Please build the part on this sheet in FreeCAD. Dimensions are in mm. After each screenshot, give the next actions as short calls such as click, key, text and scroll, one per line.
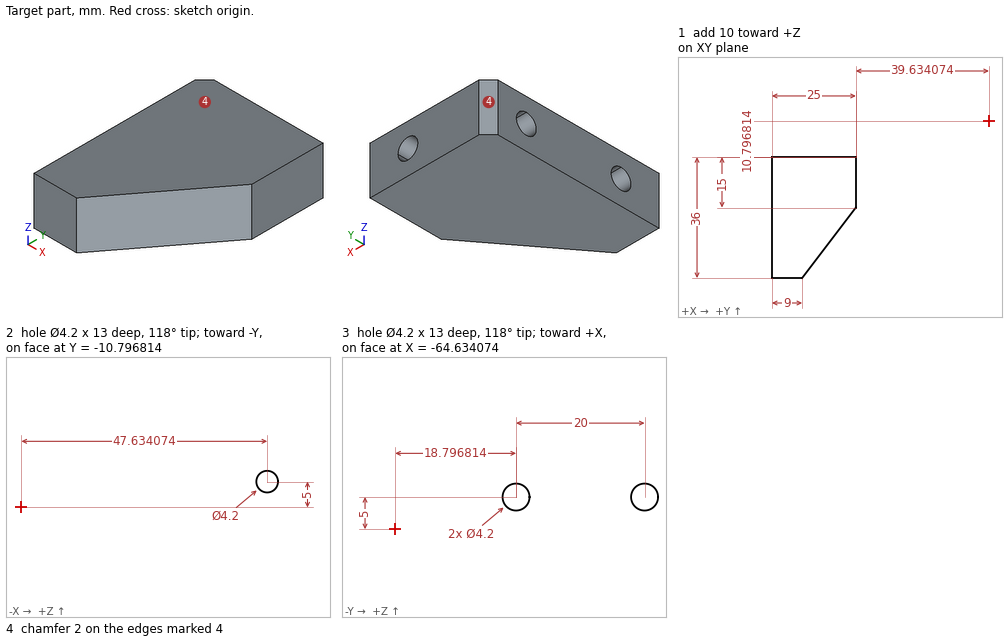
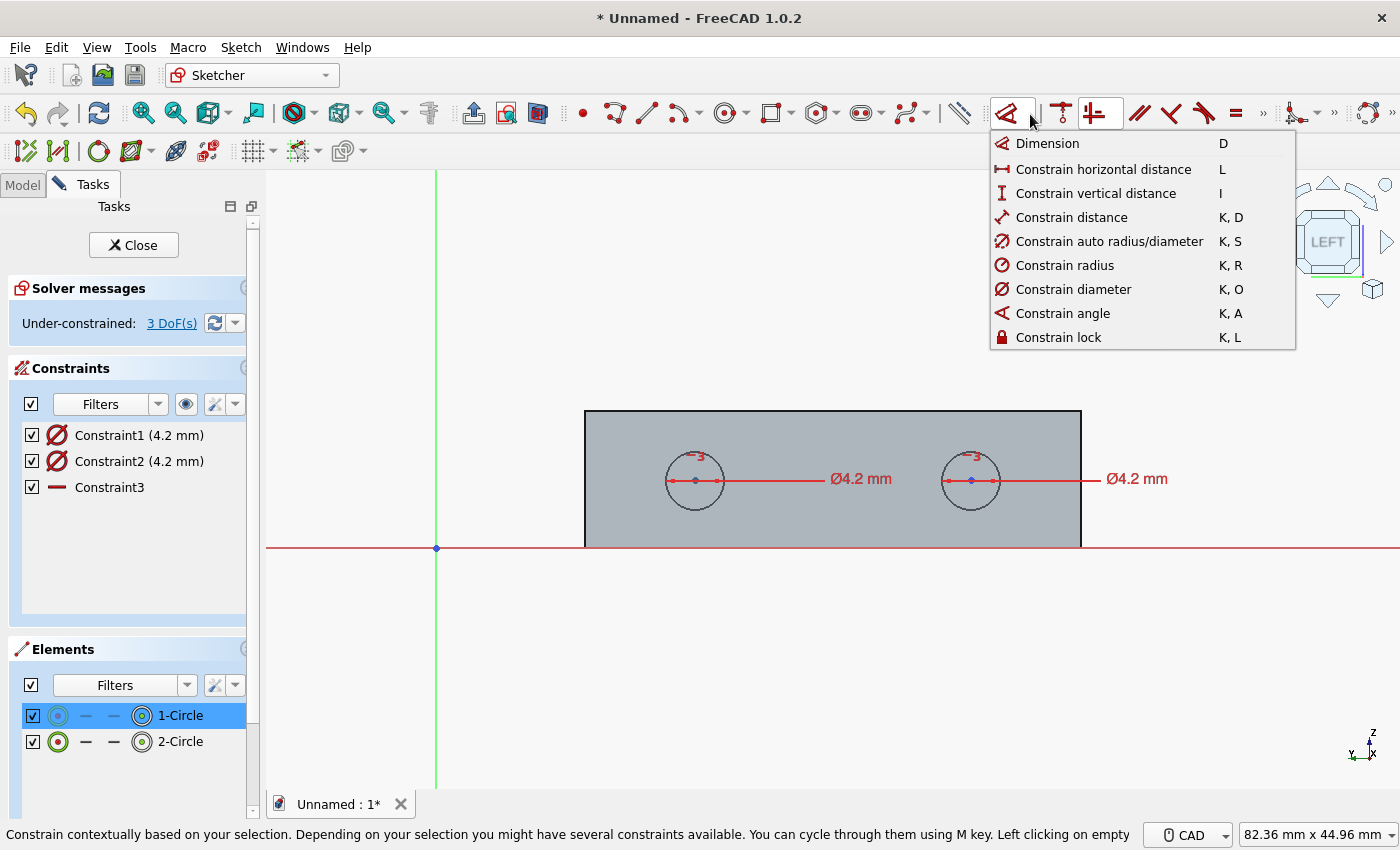
click(1143, 193)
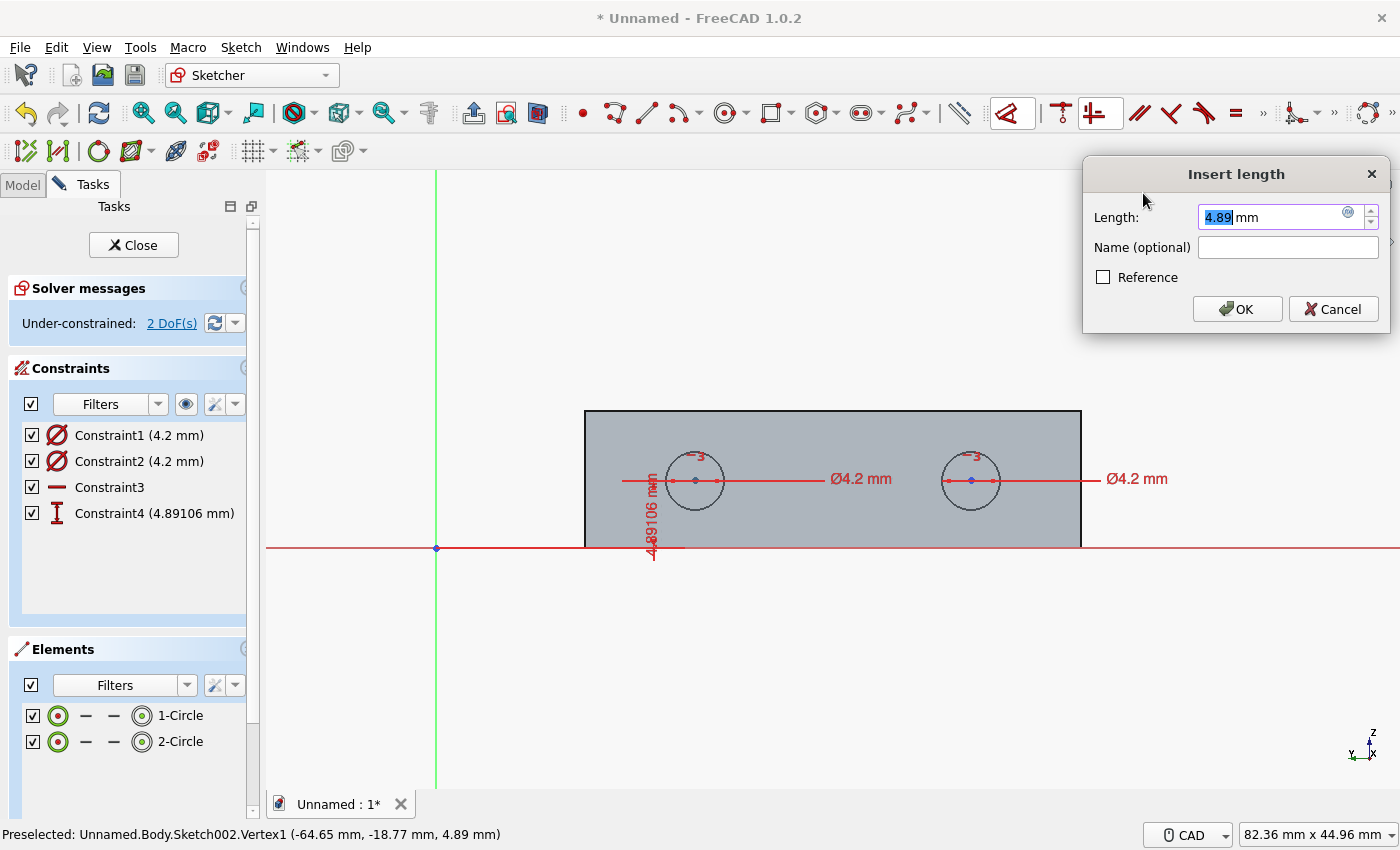
text(5)
key(Return)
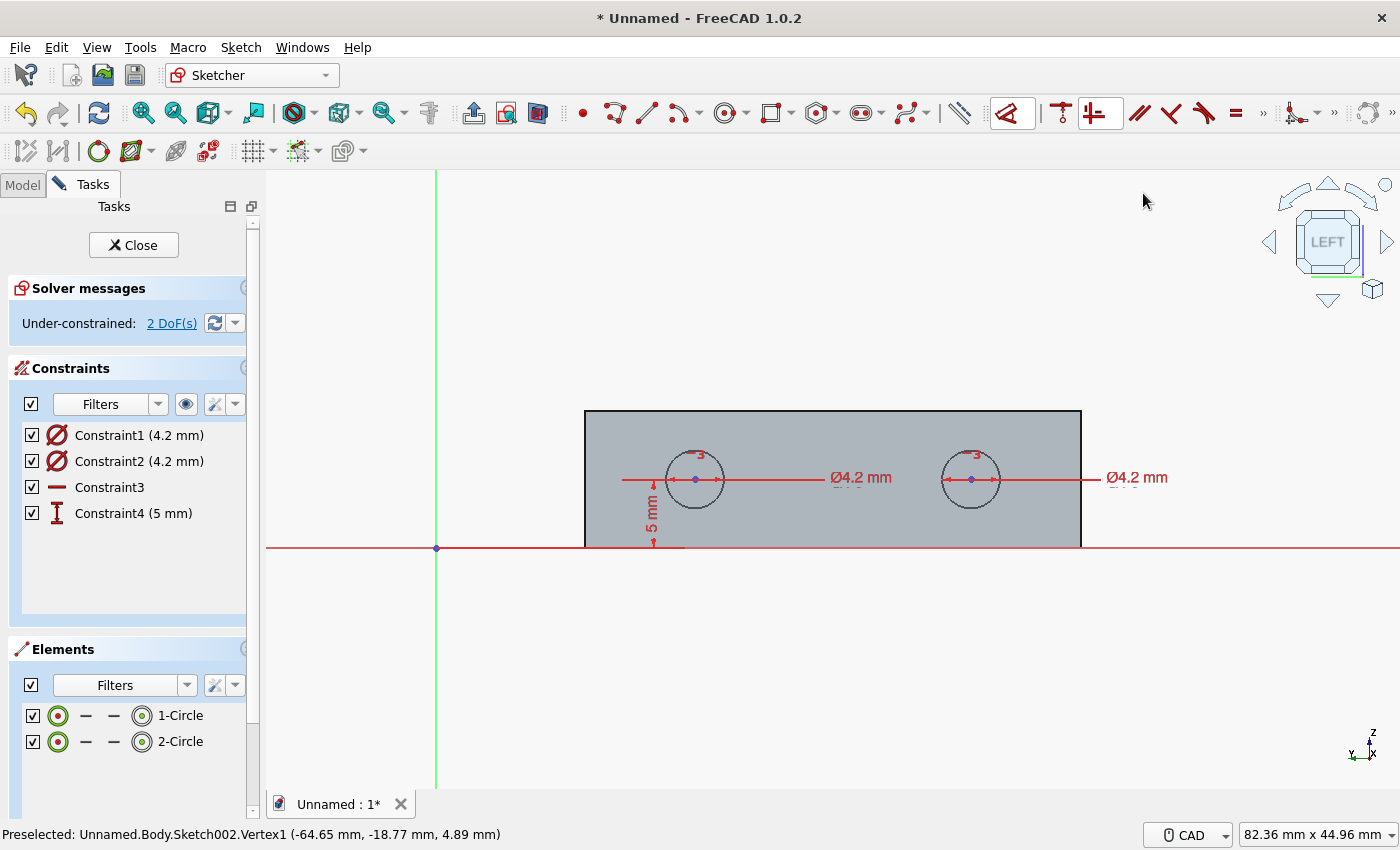
click(695, 480)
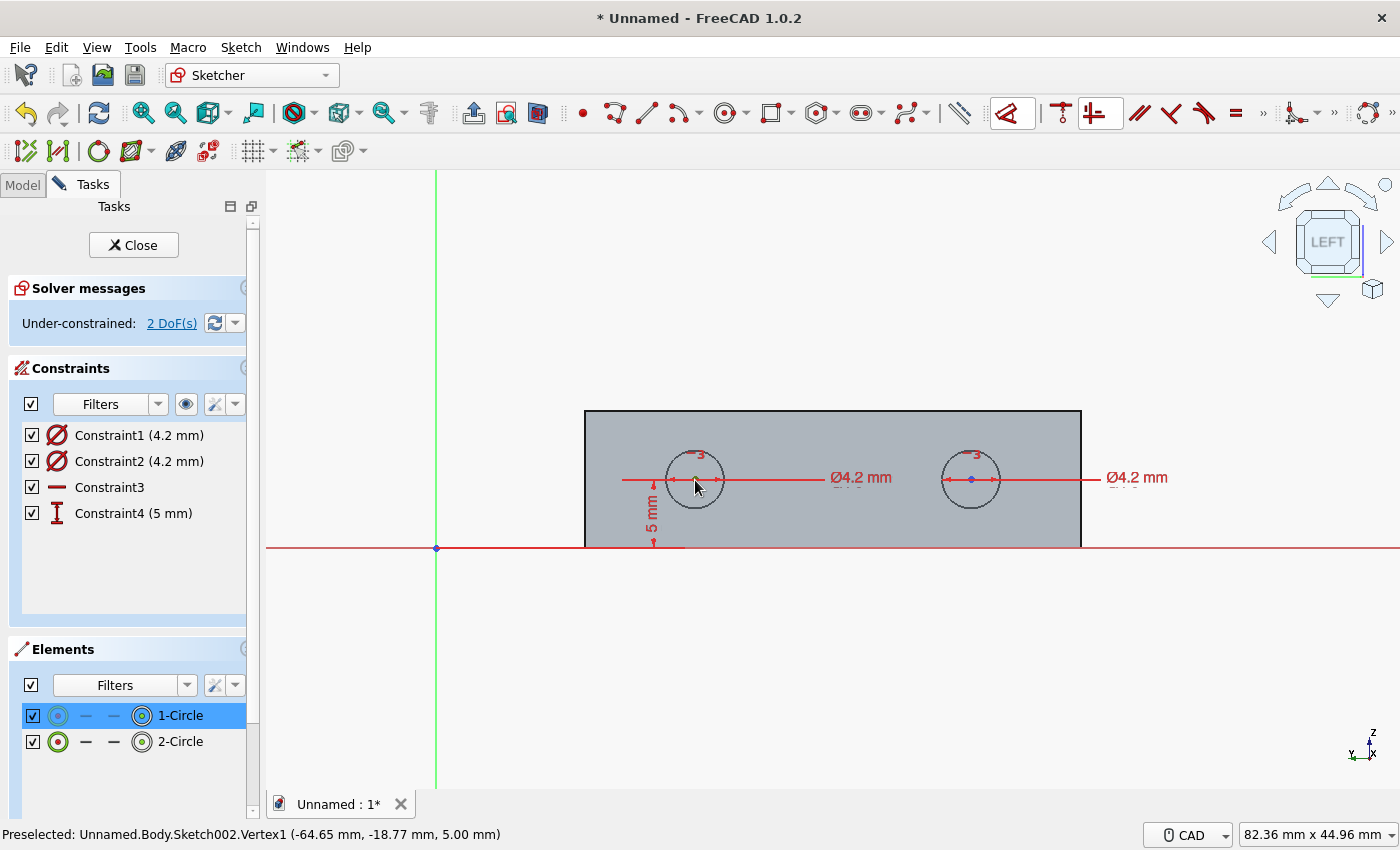
click(971, 480)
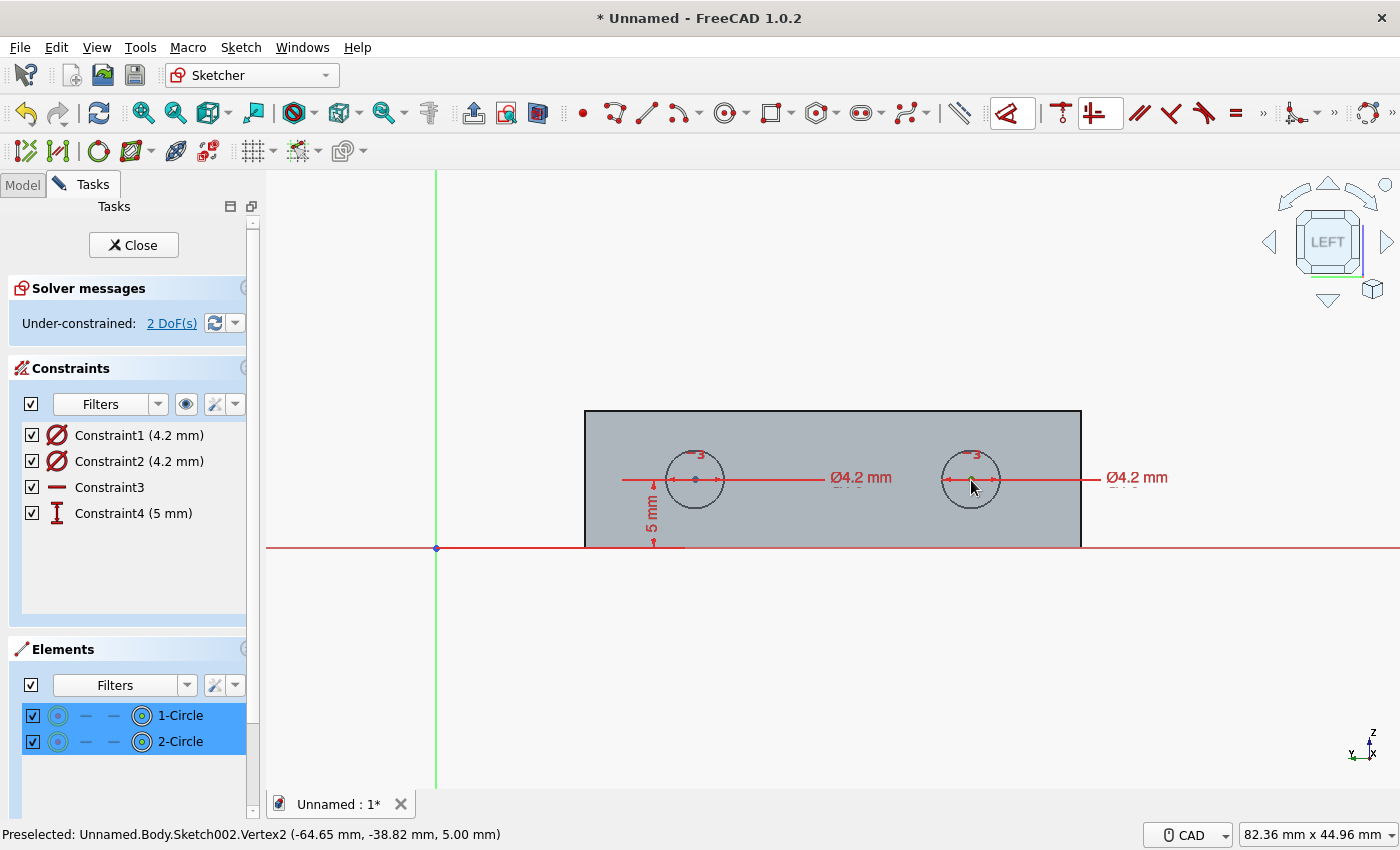
click(1030, 114)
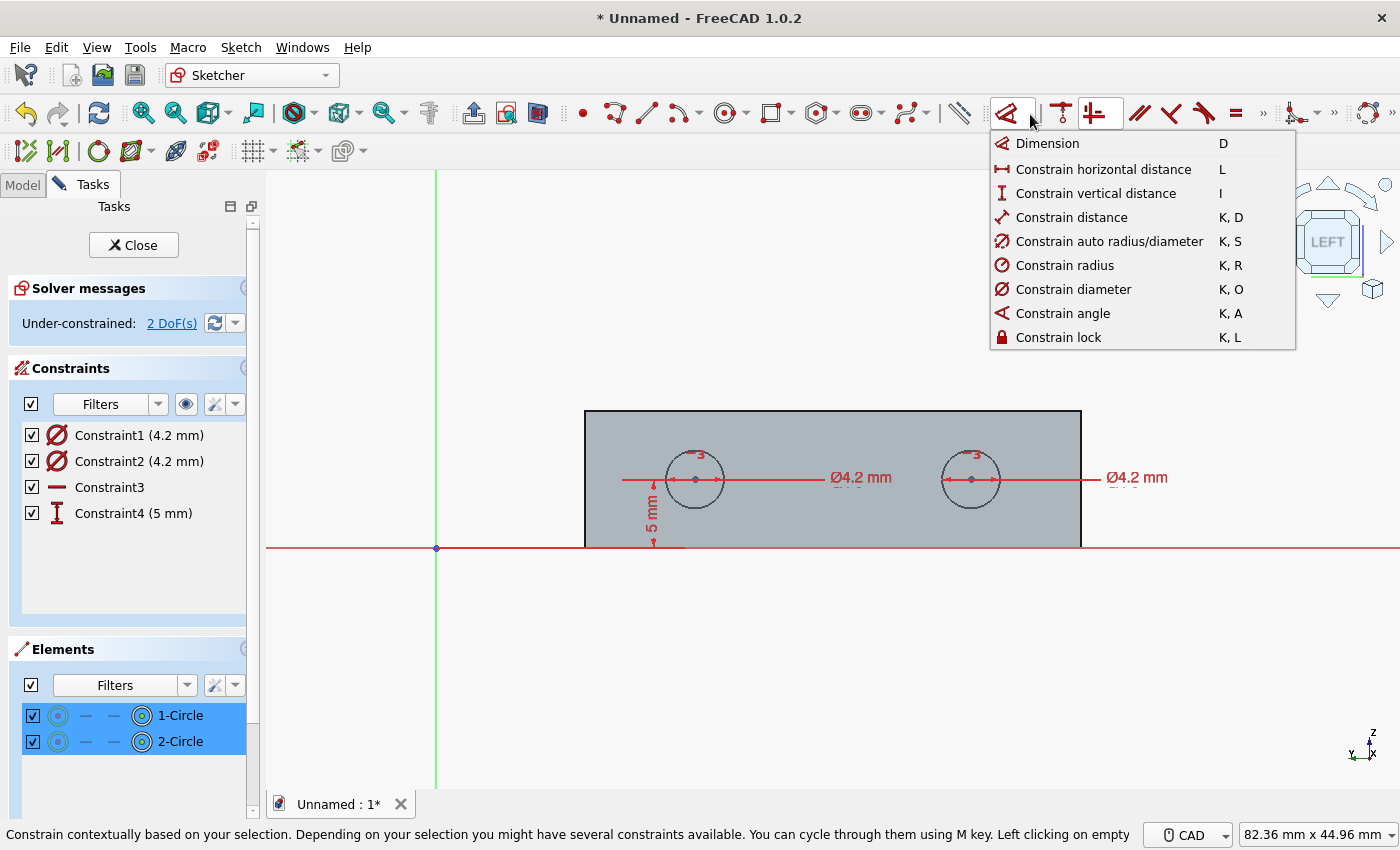
click(1143, 169)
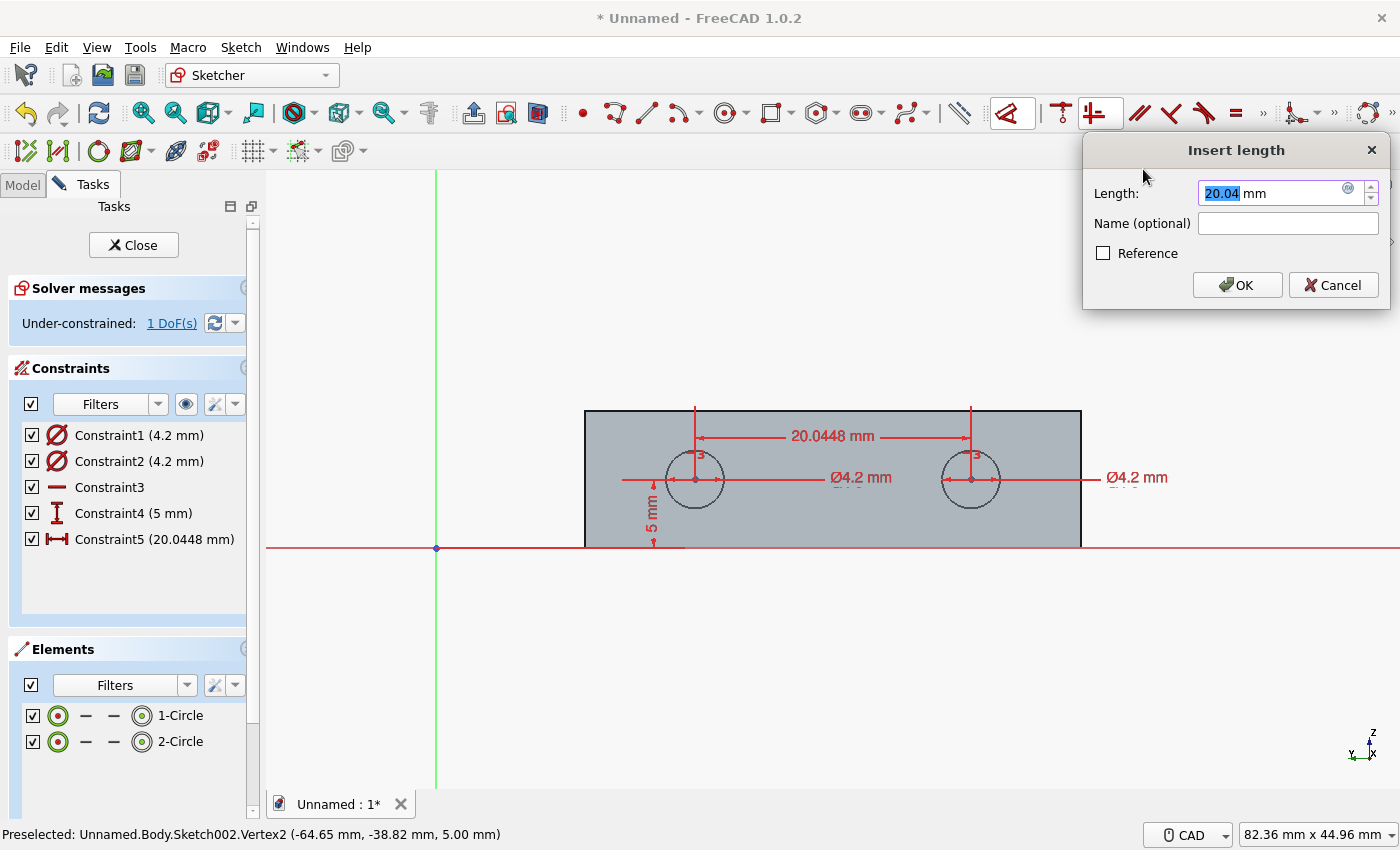
text(20)
key(Return)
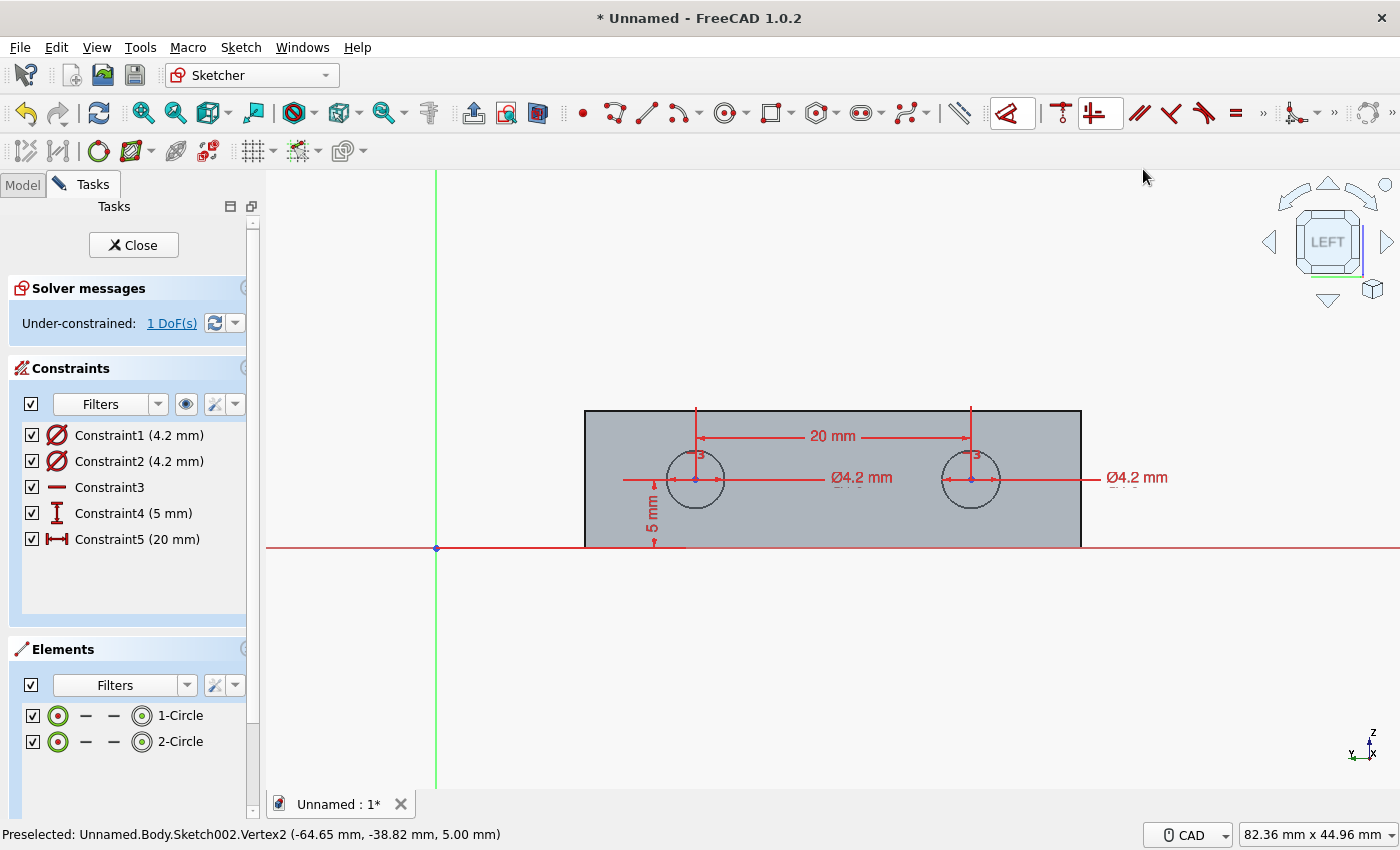
click(696, 480)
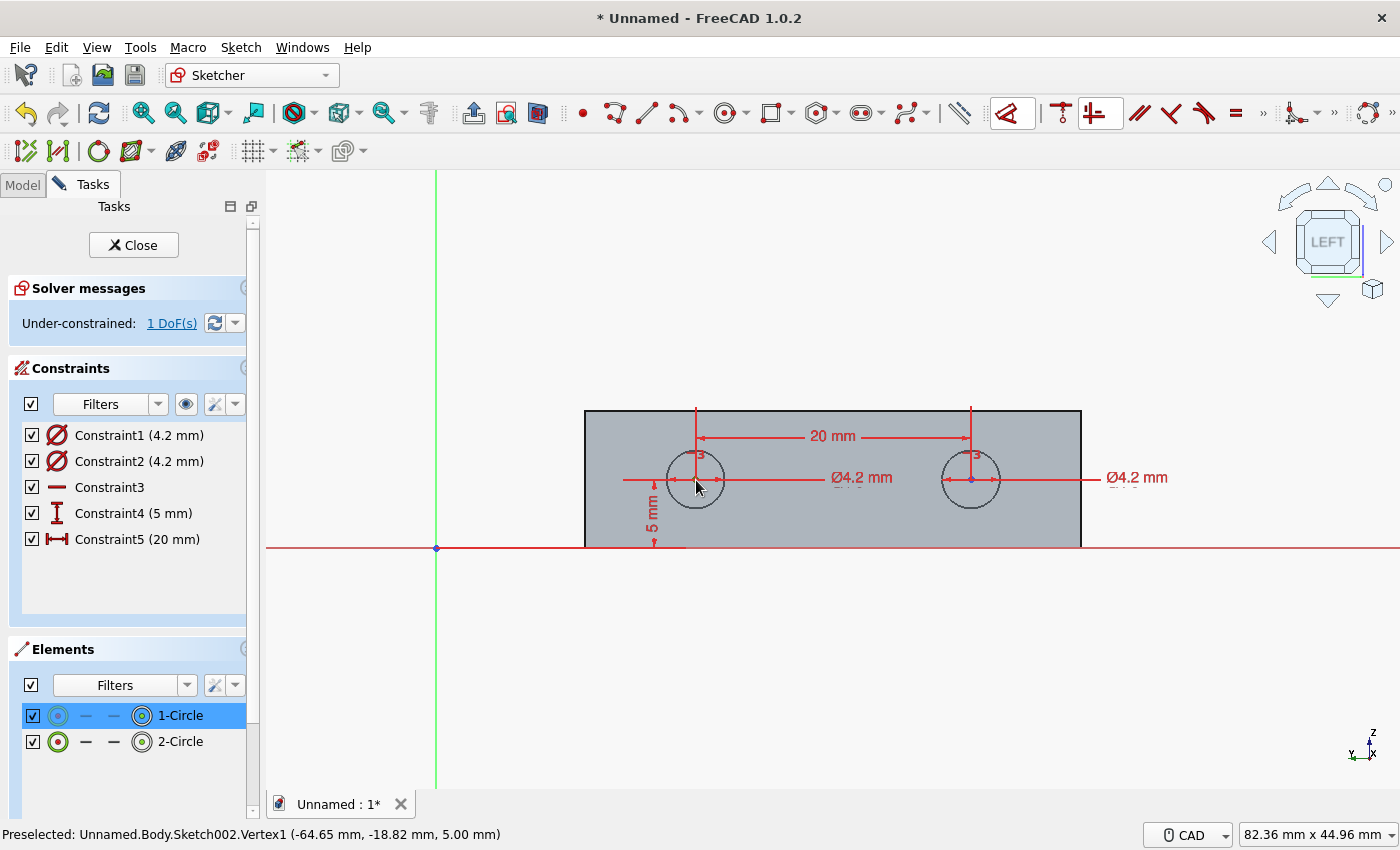
click(1030, 114)